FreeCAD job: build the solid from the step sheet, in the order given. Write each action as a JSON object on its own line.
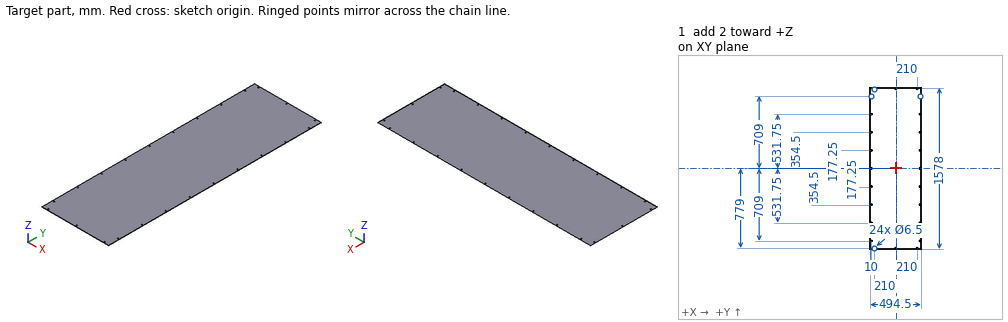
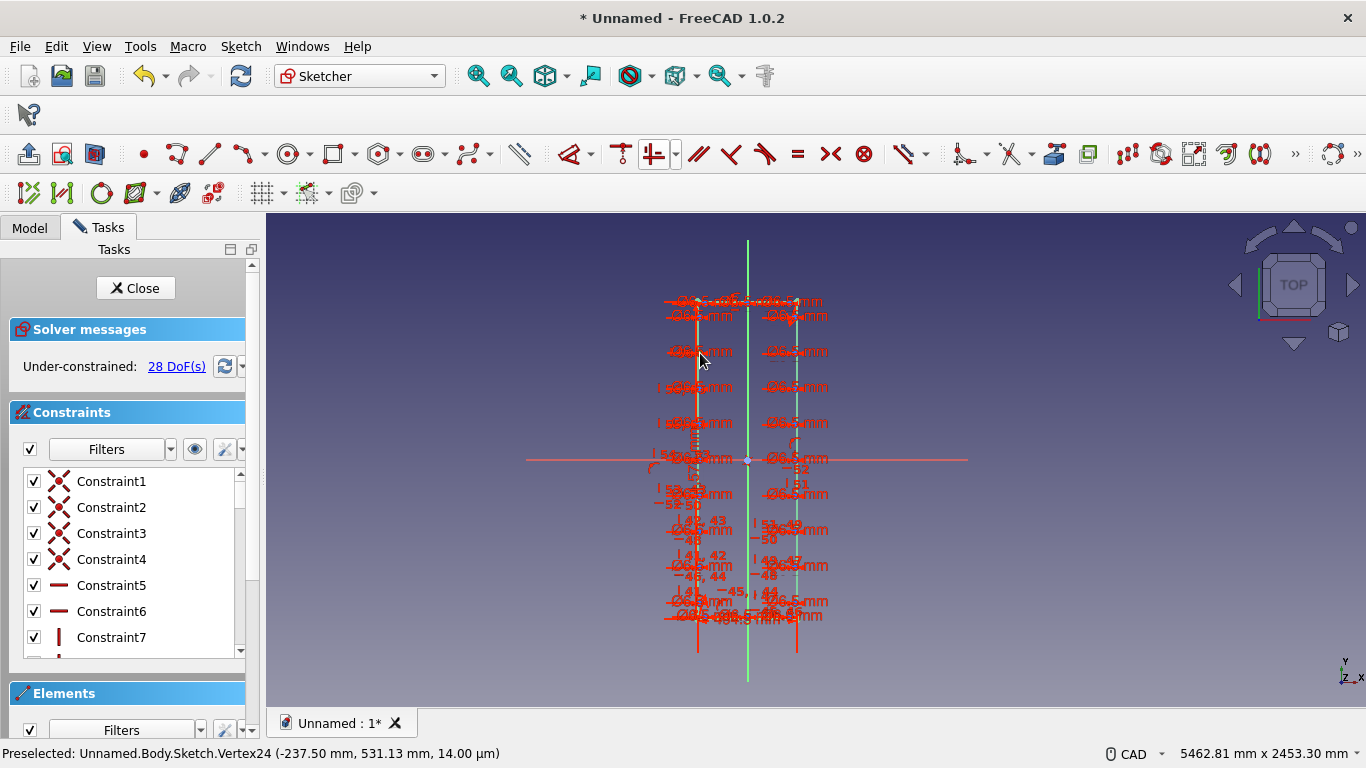
{"action": "left_click", "coordinate": [700, 318]}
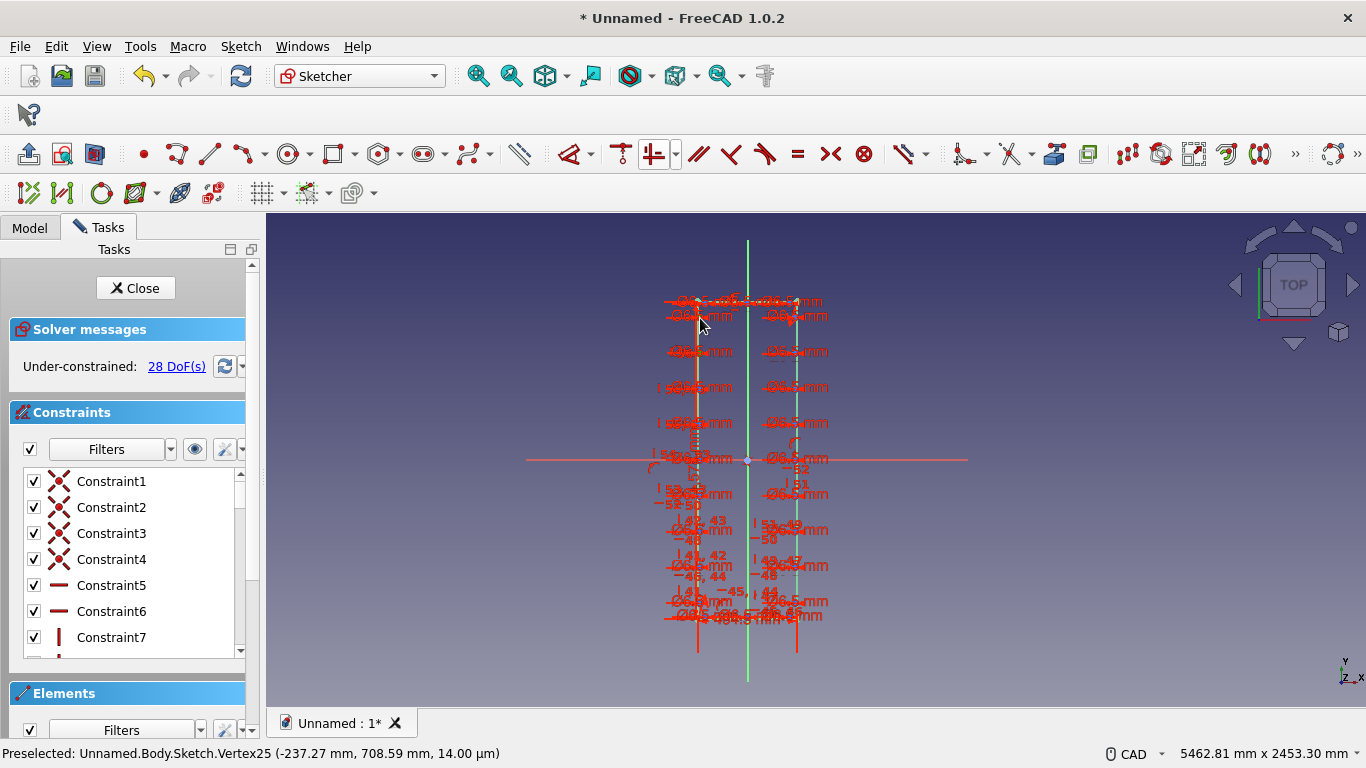
{"action": "left_click", "coordinate": [676, 154]}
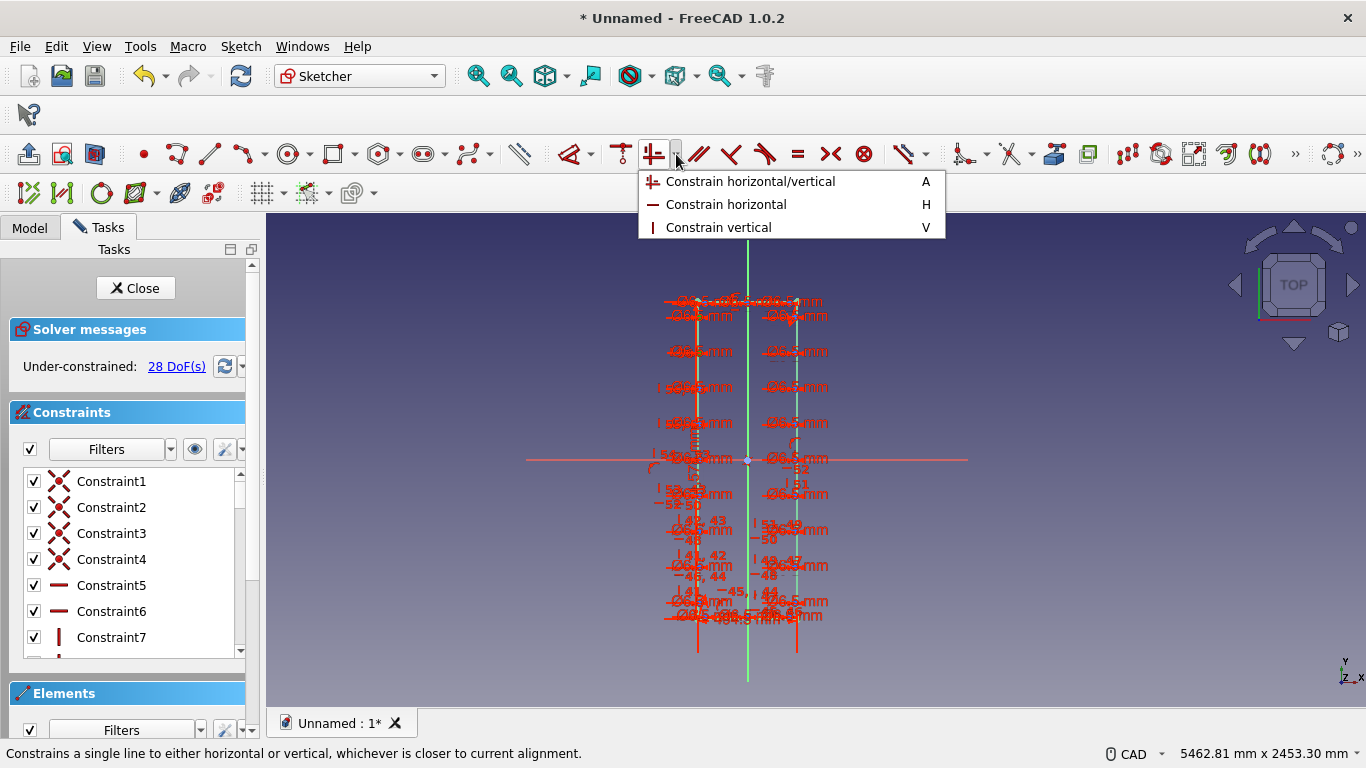
{"action": "left_click", "coordinate": [792, 228]}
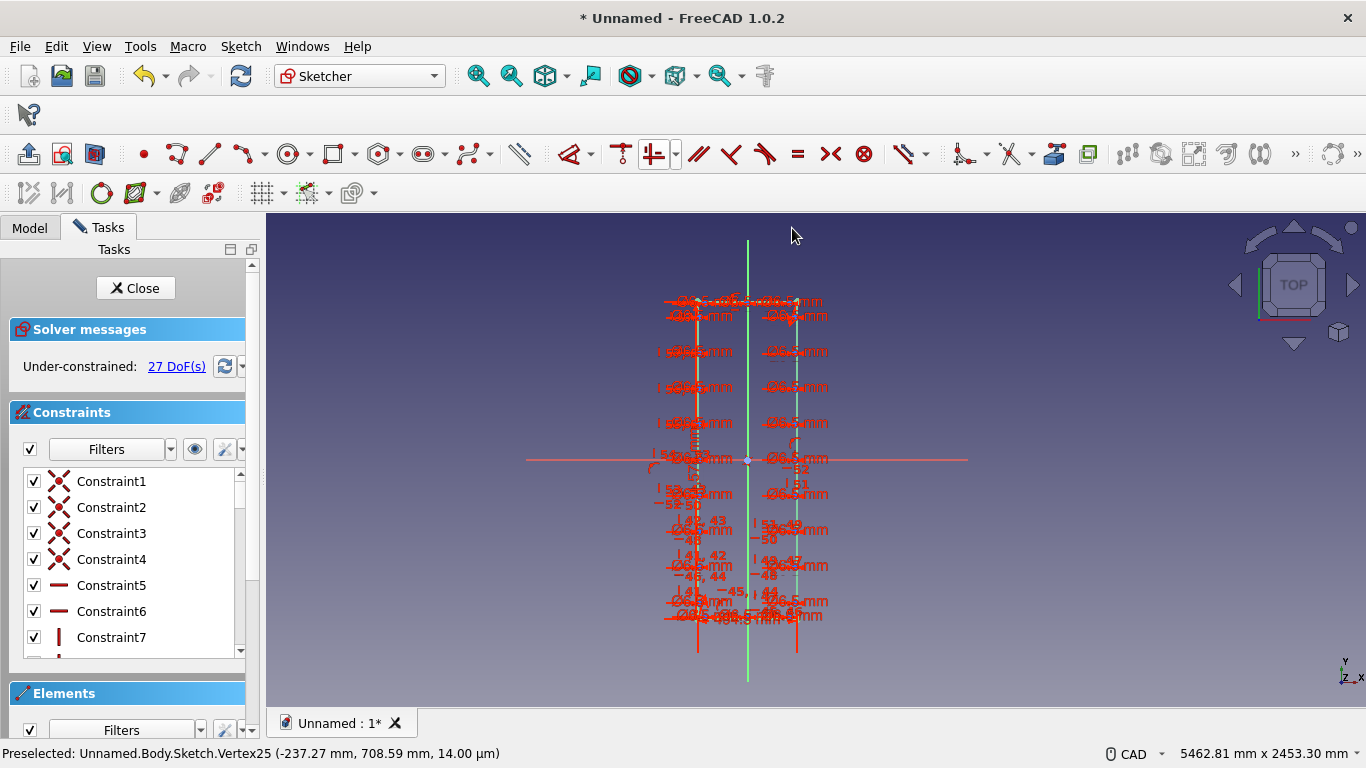
{"action": "left_click", "coordinate": [795, 496]}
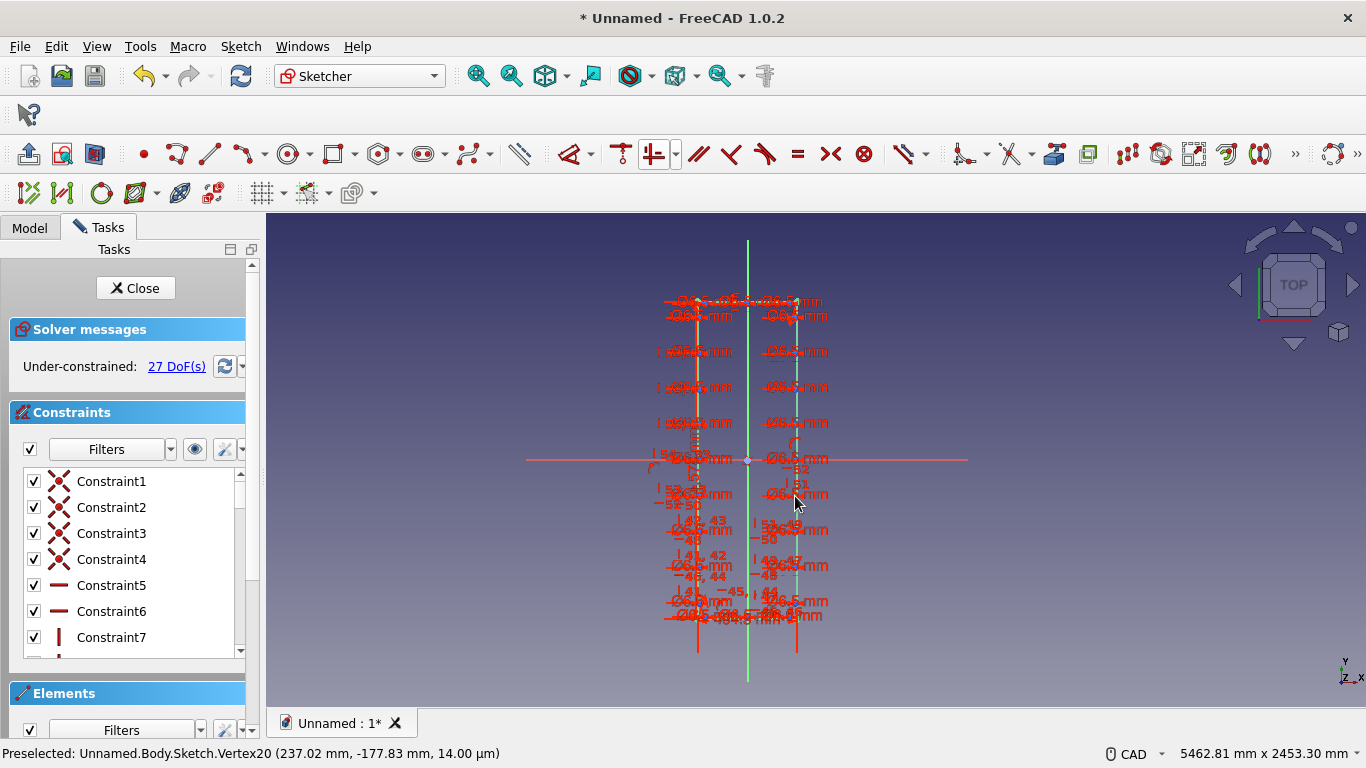
{"action": "left_click", "coordinate": [795, 460]}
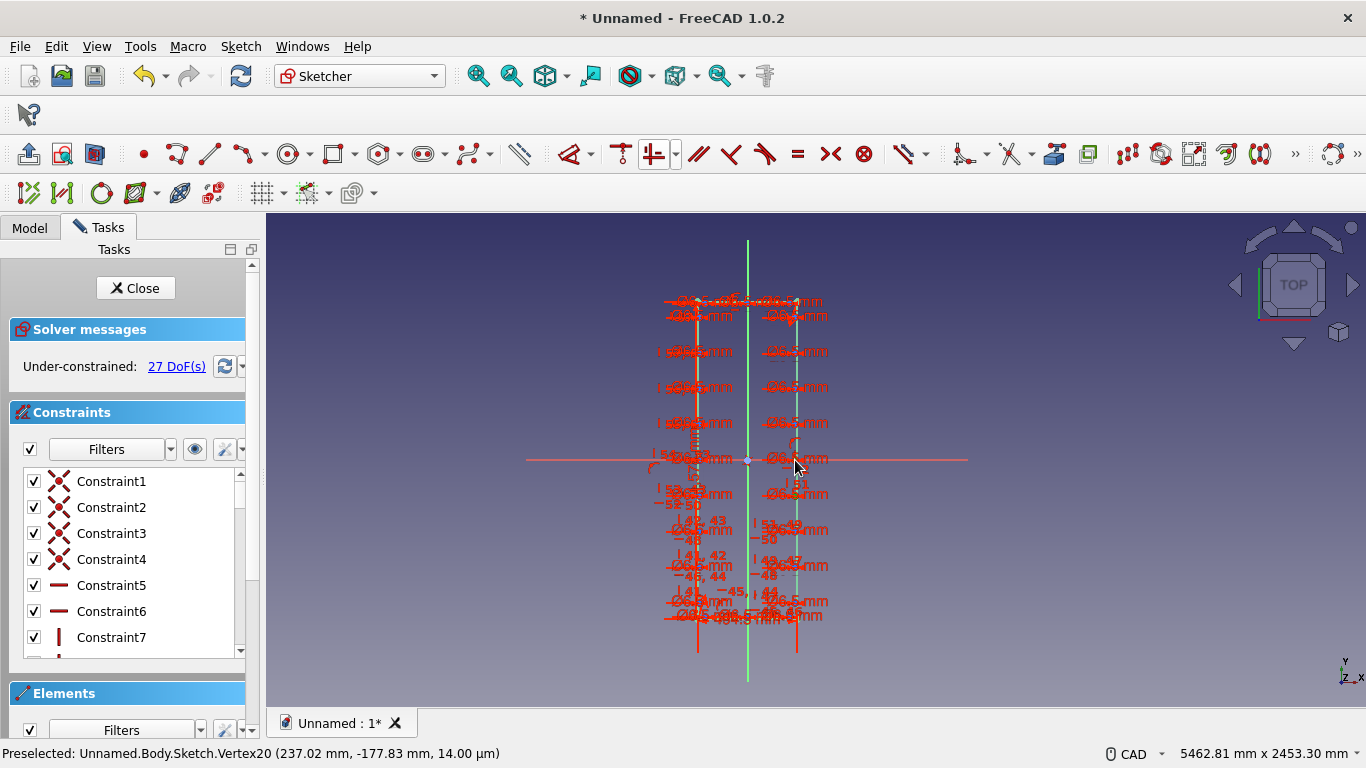
{"action": "key", "text": "v"}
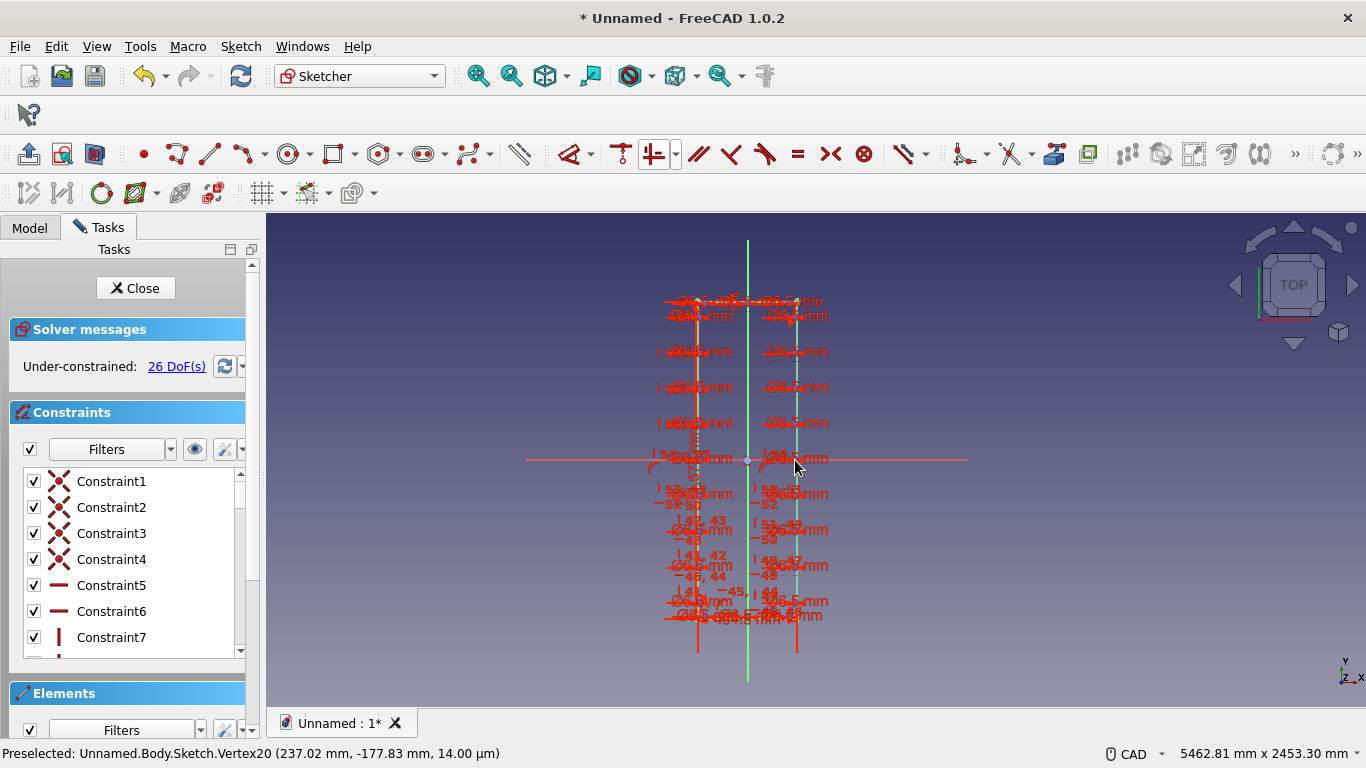
{"action": "left_click", "coordinate": [795, 460]}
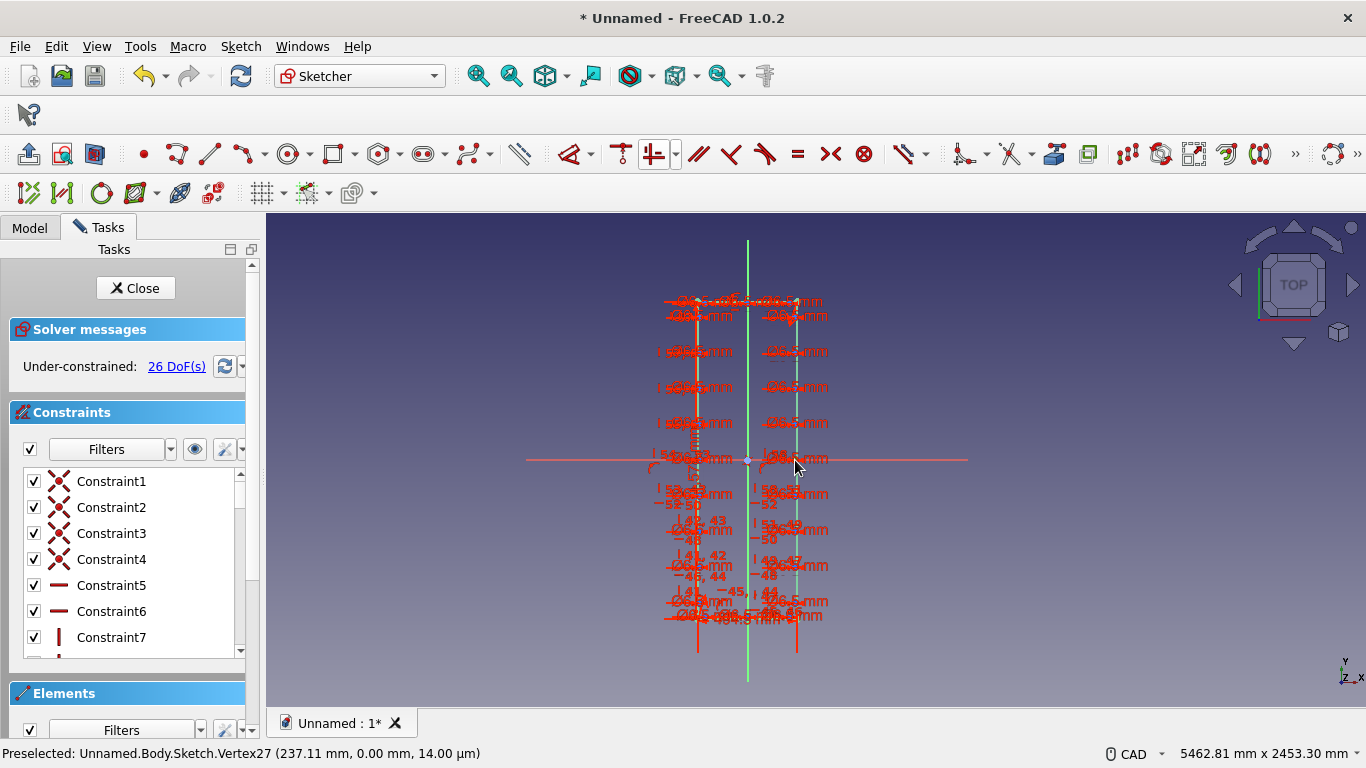
{"action": "left_click", "coordinate": [795, 425]}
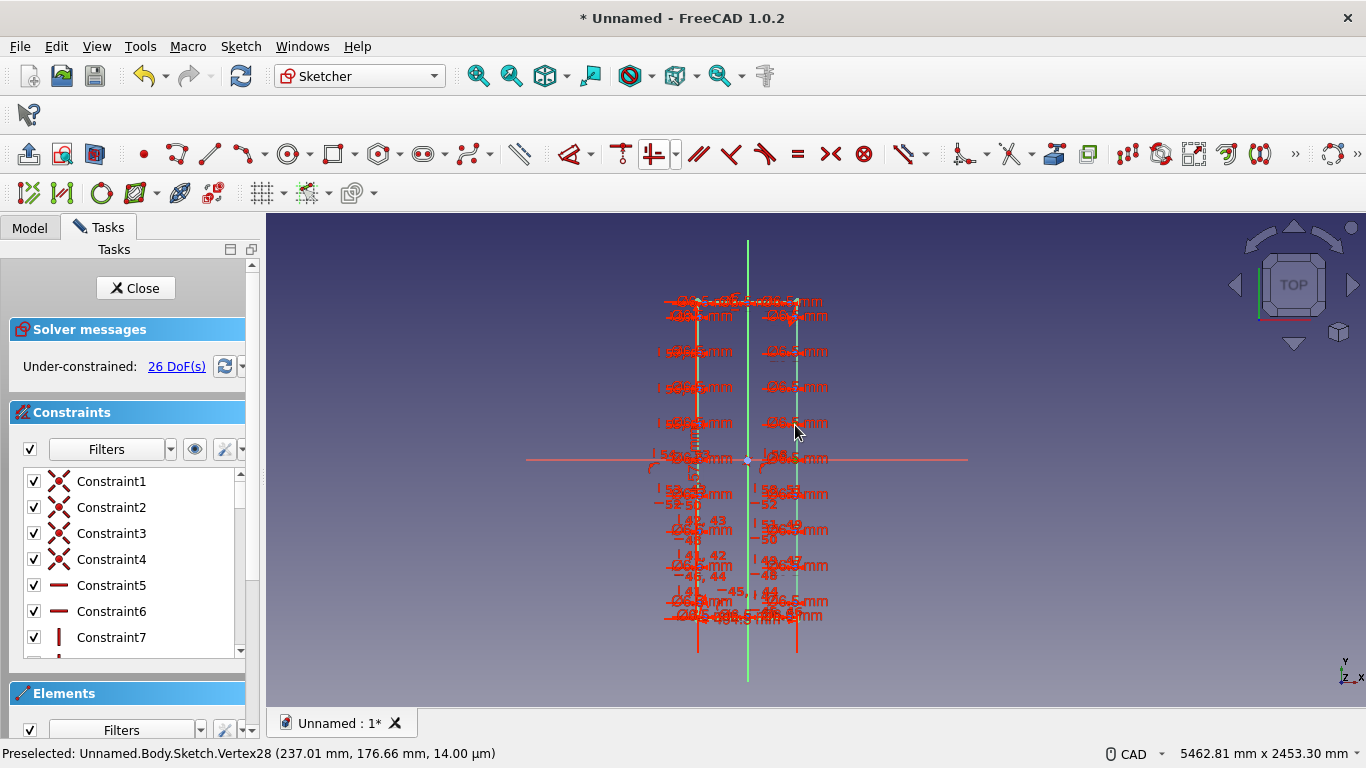
{"action": "key", "text": "v"}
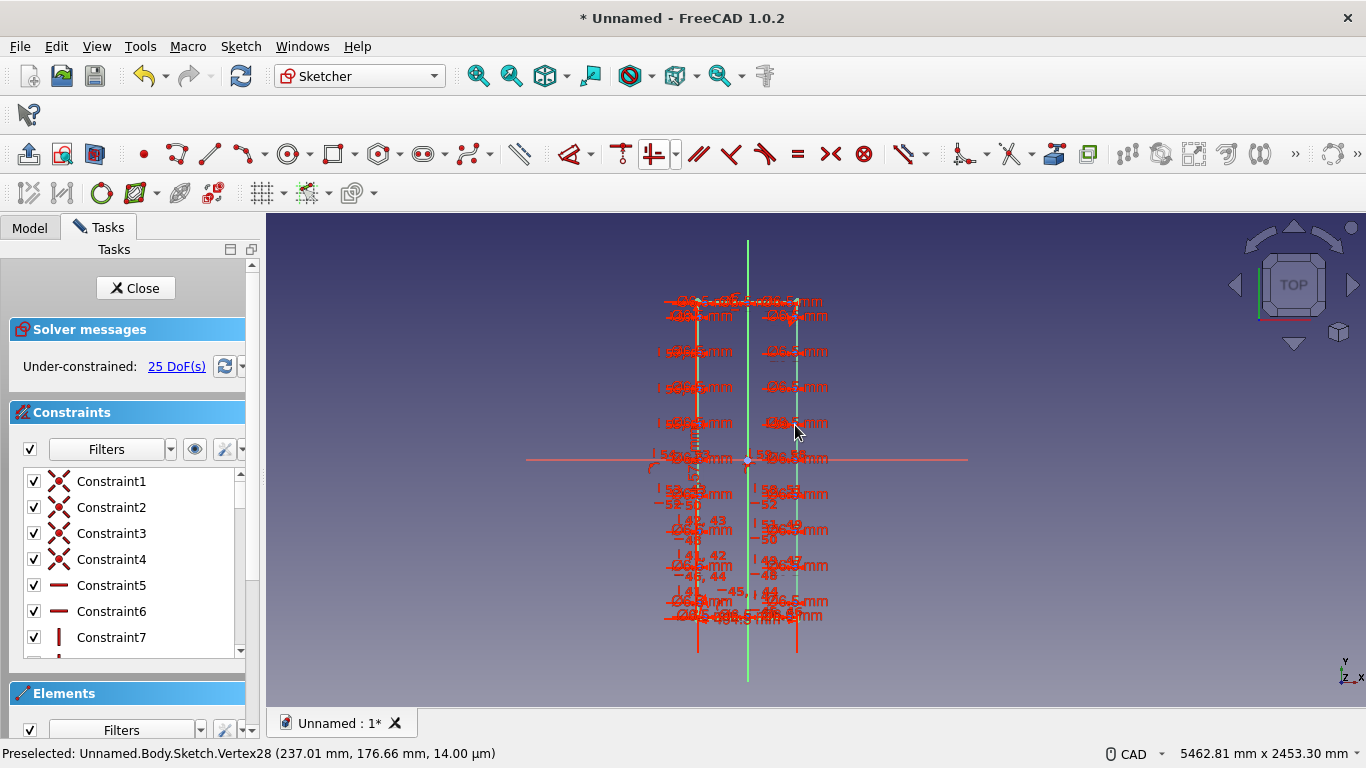
{"action": "left_click", "coordinate": [700, 425]}